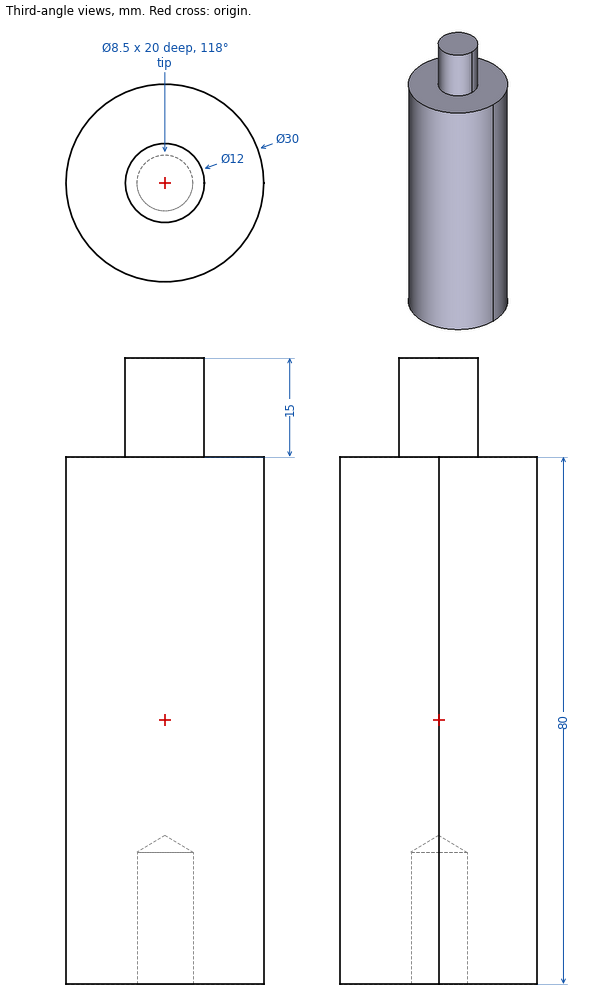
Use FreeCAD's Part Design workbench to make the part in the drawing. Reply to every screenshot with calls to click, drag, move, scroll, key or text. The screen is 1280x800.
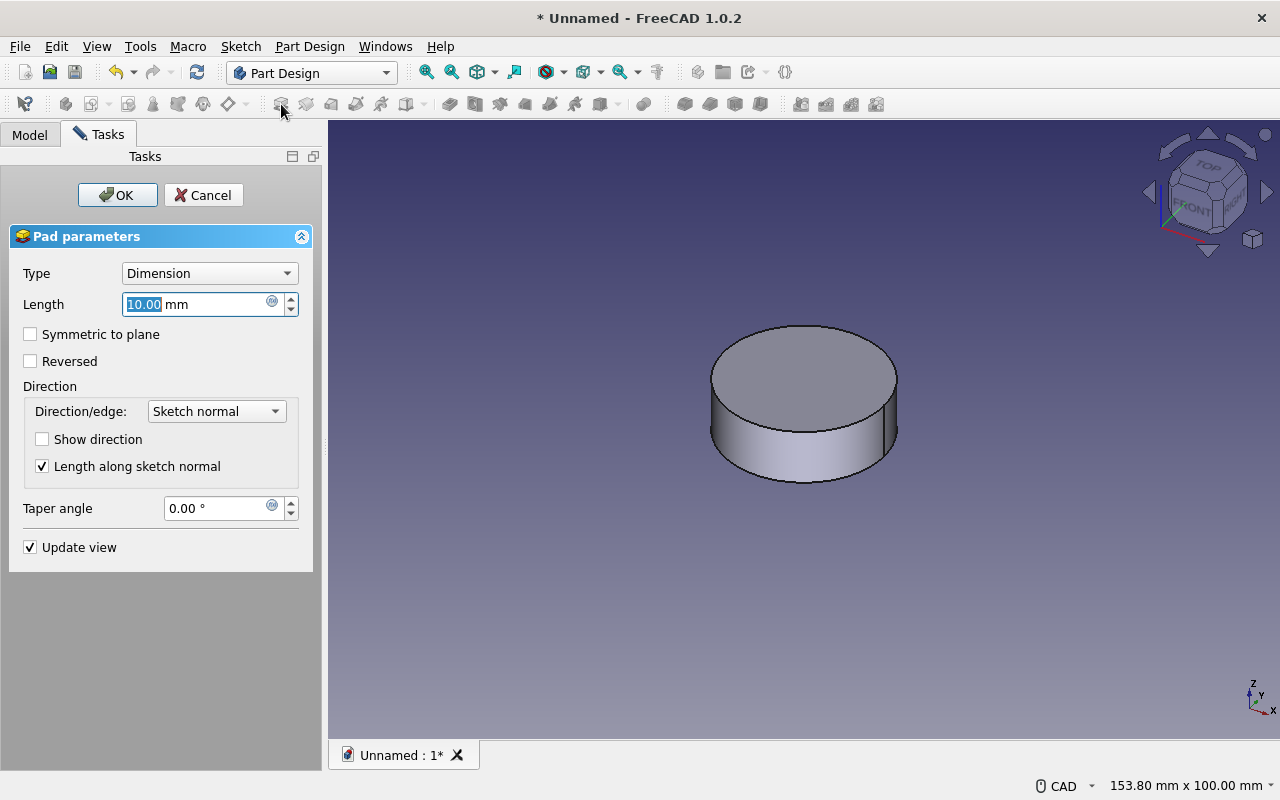
text(80)
key(Tab)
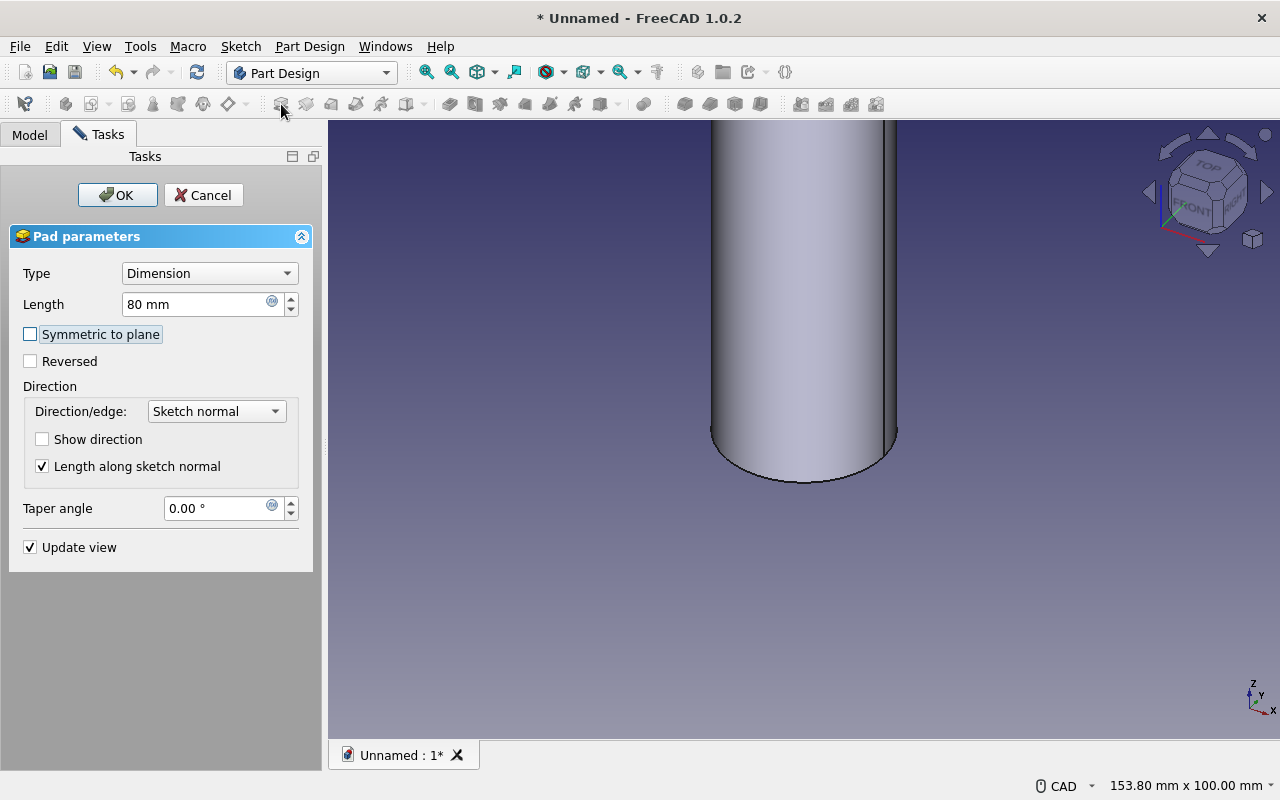
click(31, 334)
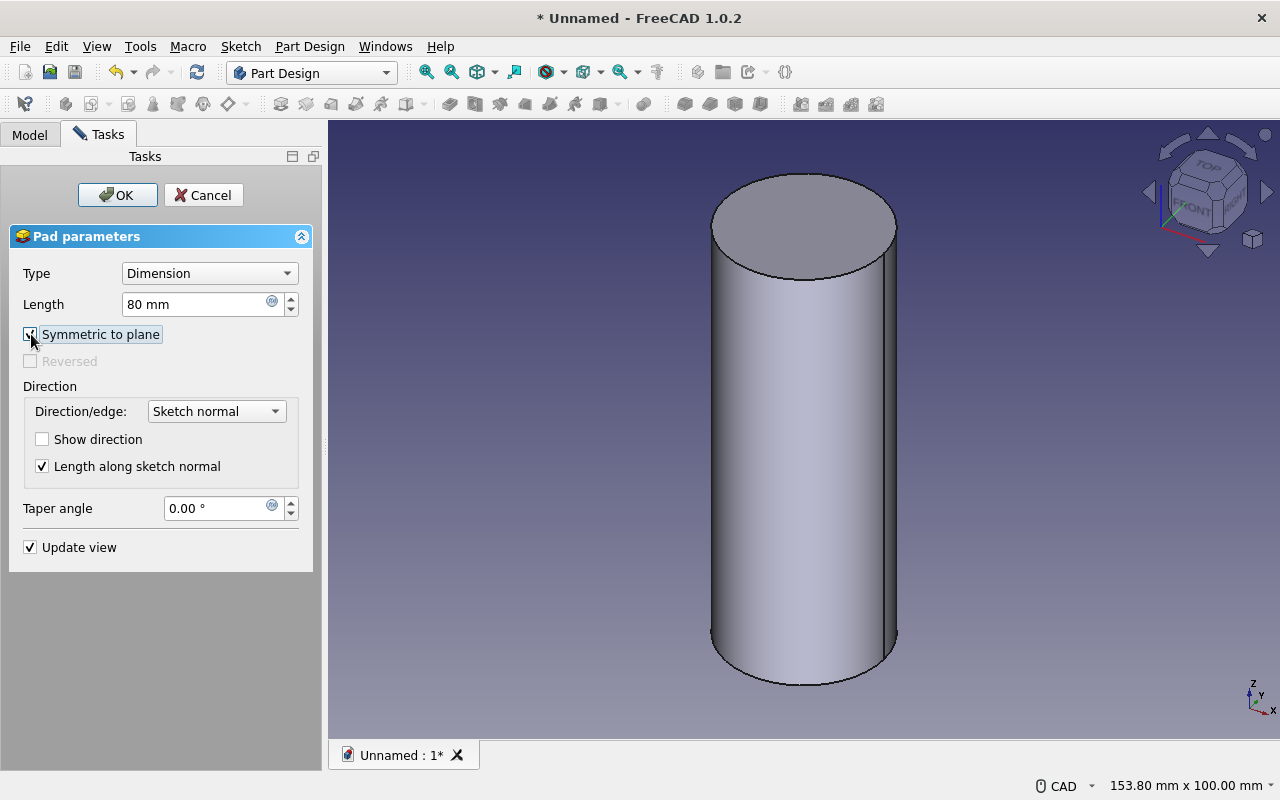
click(118, 195)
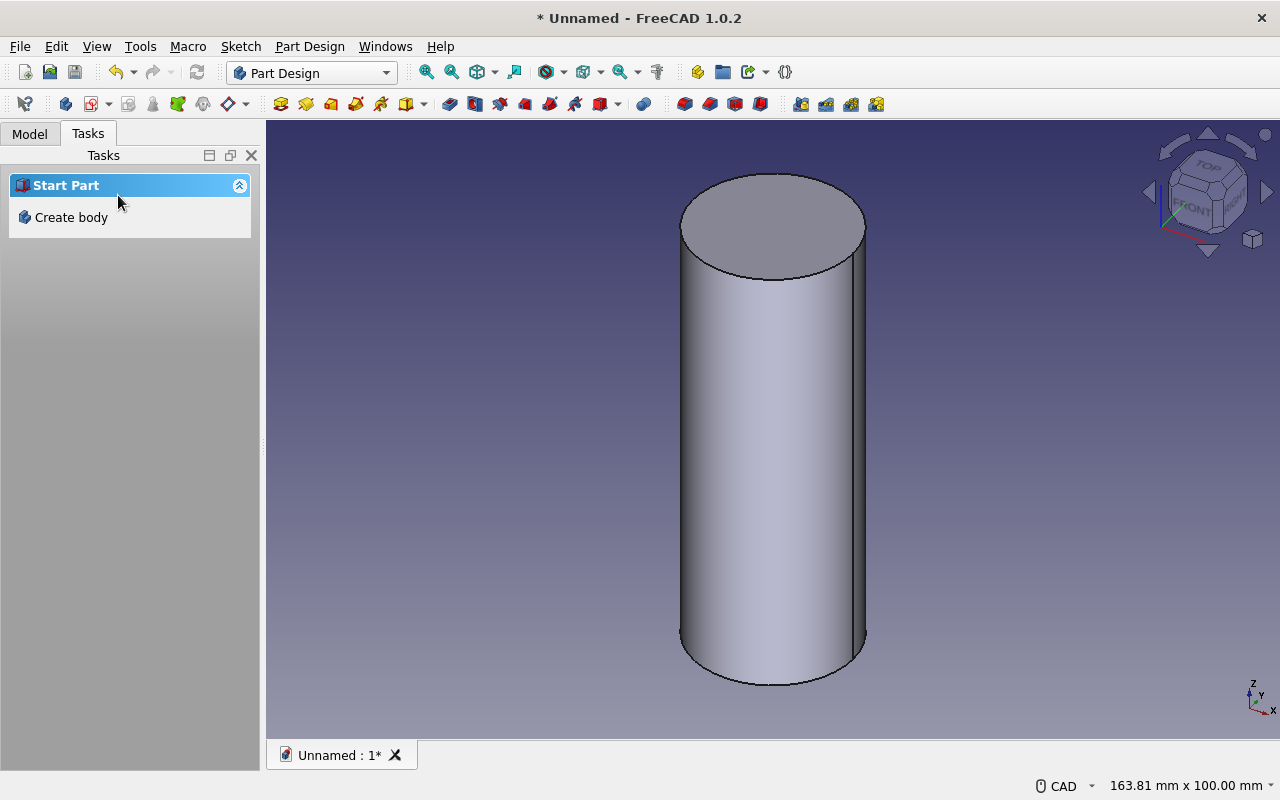
key(5)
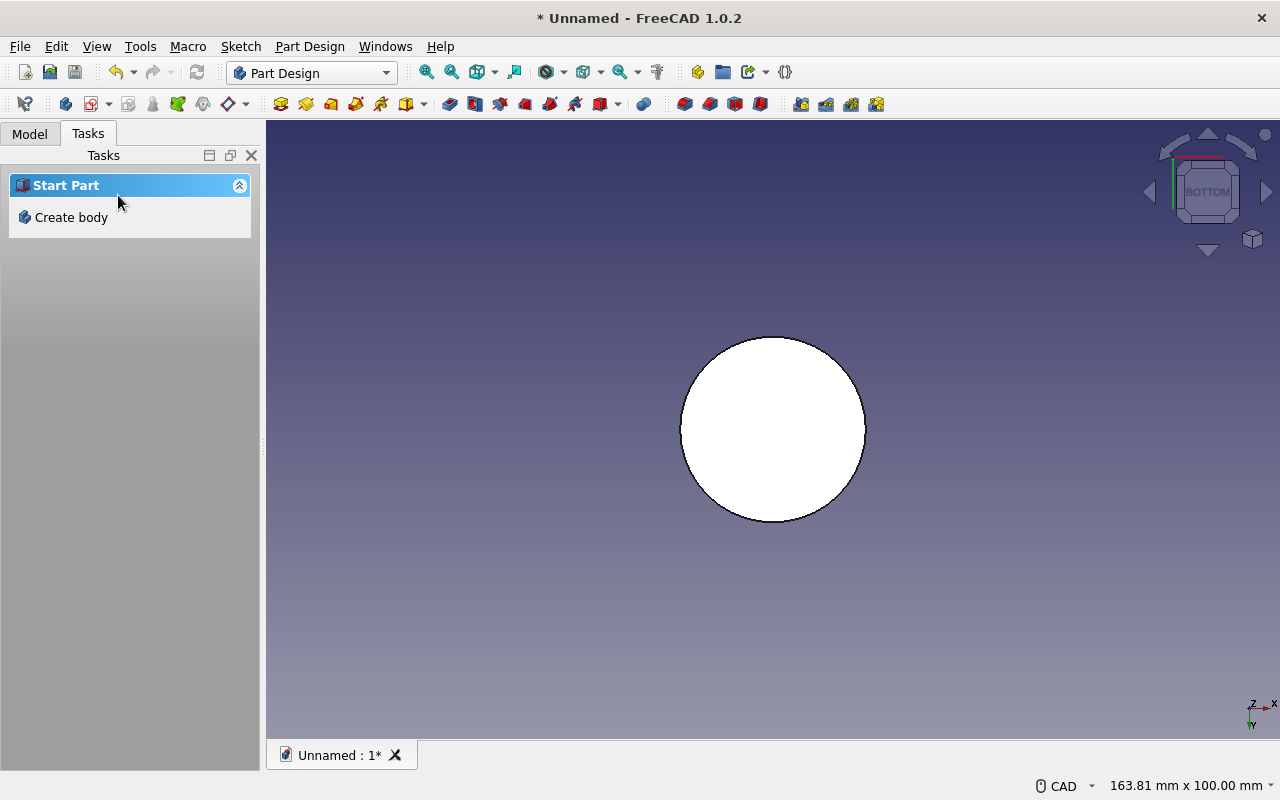
click(427, 72)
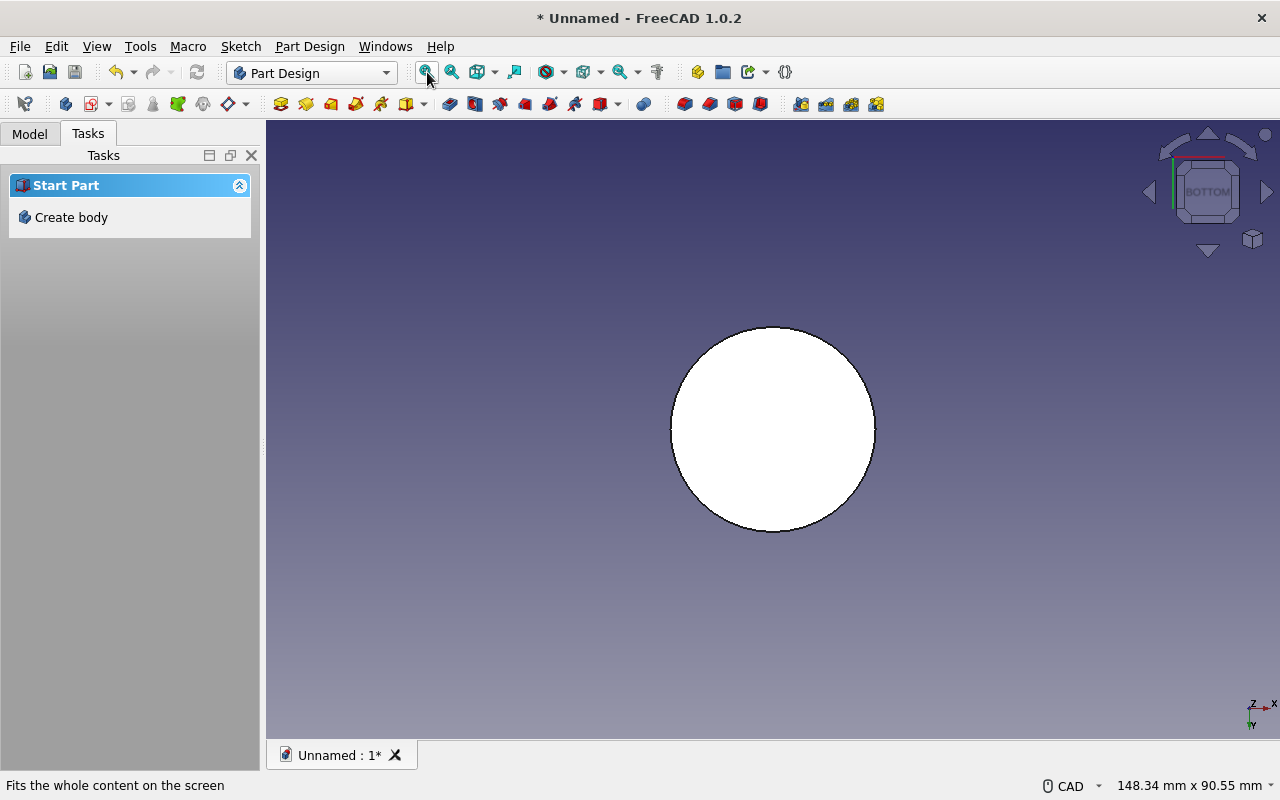
click(773, 428)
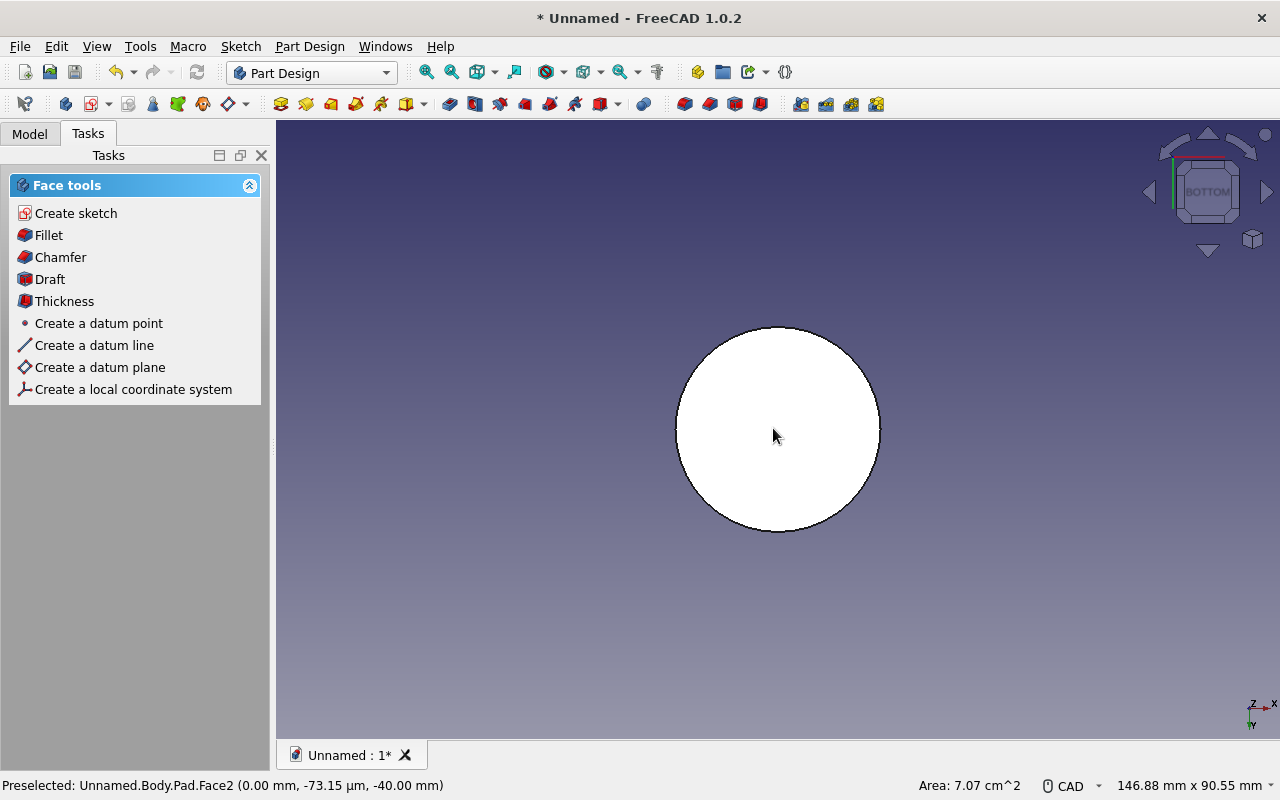
click(90, 104)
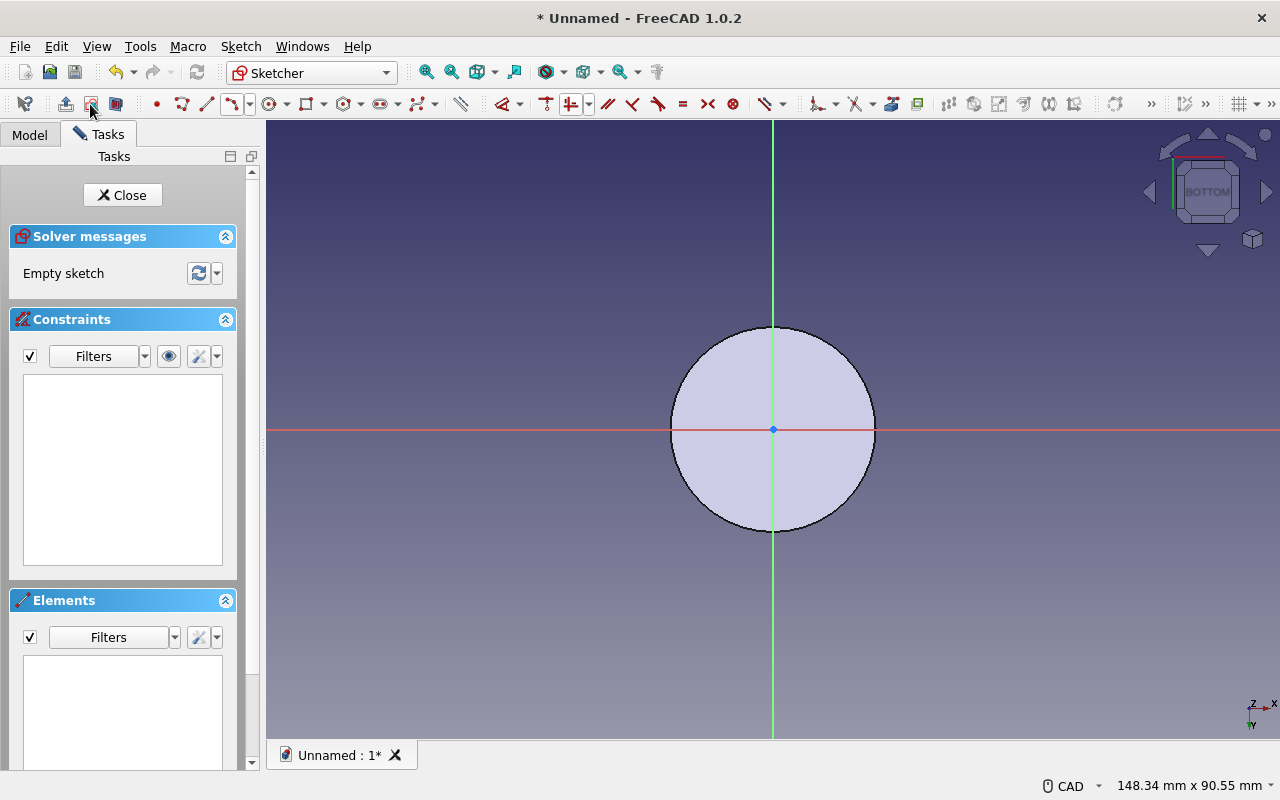
scroll(784, 430, up, 10)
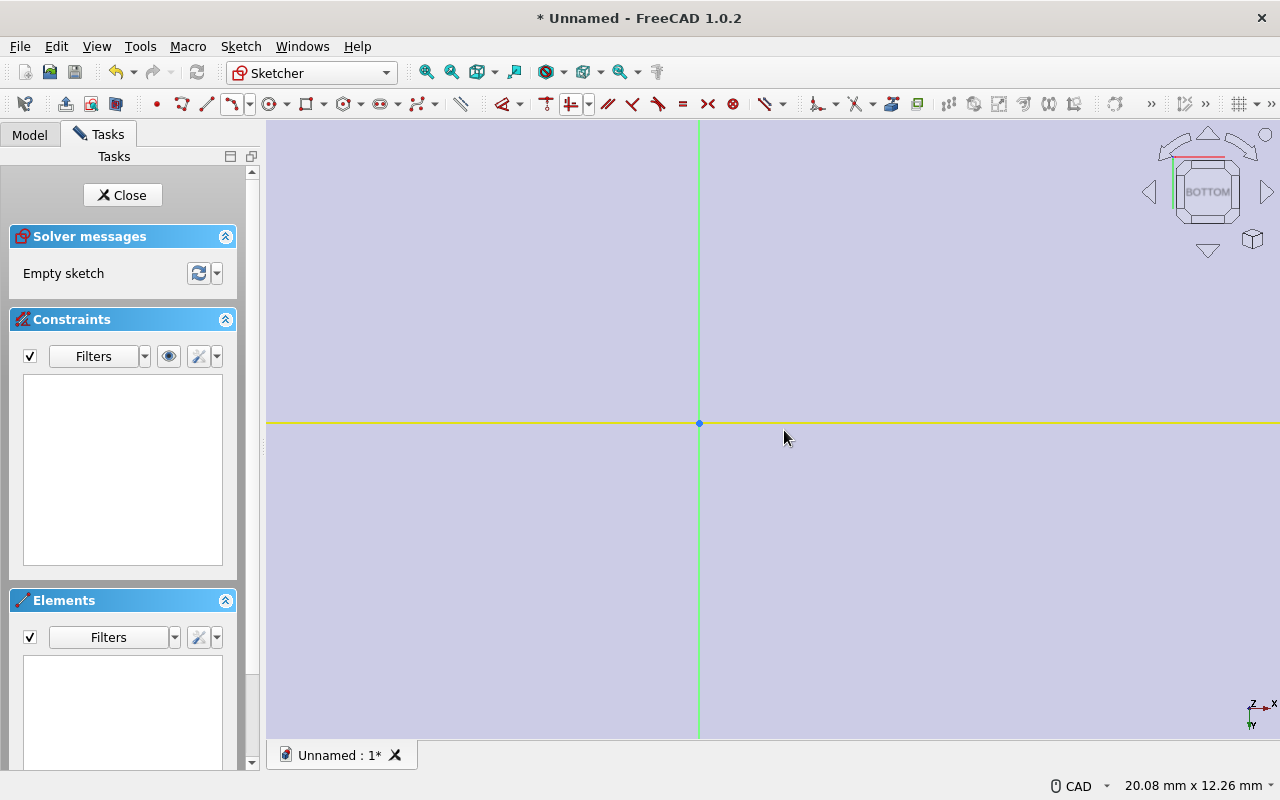
click(268, 104)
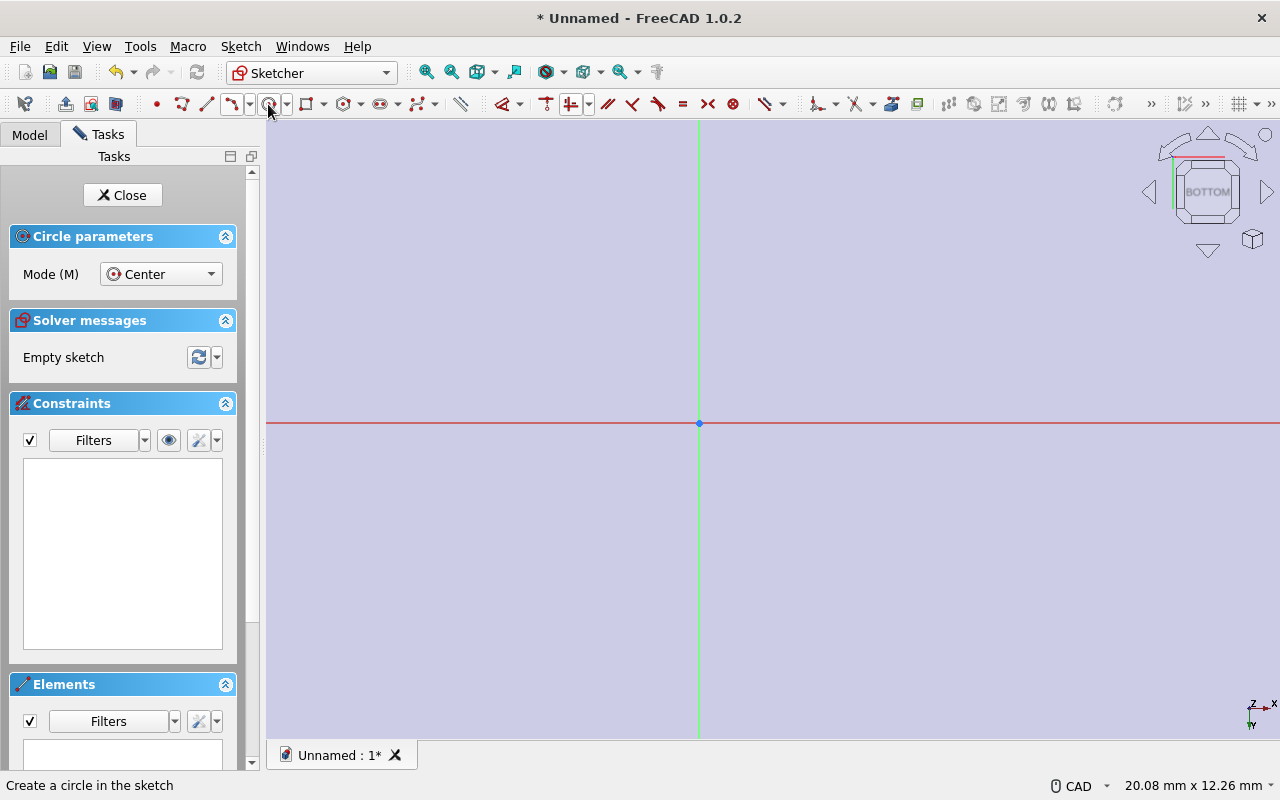
click(699, 423)
move(851, 271)